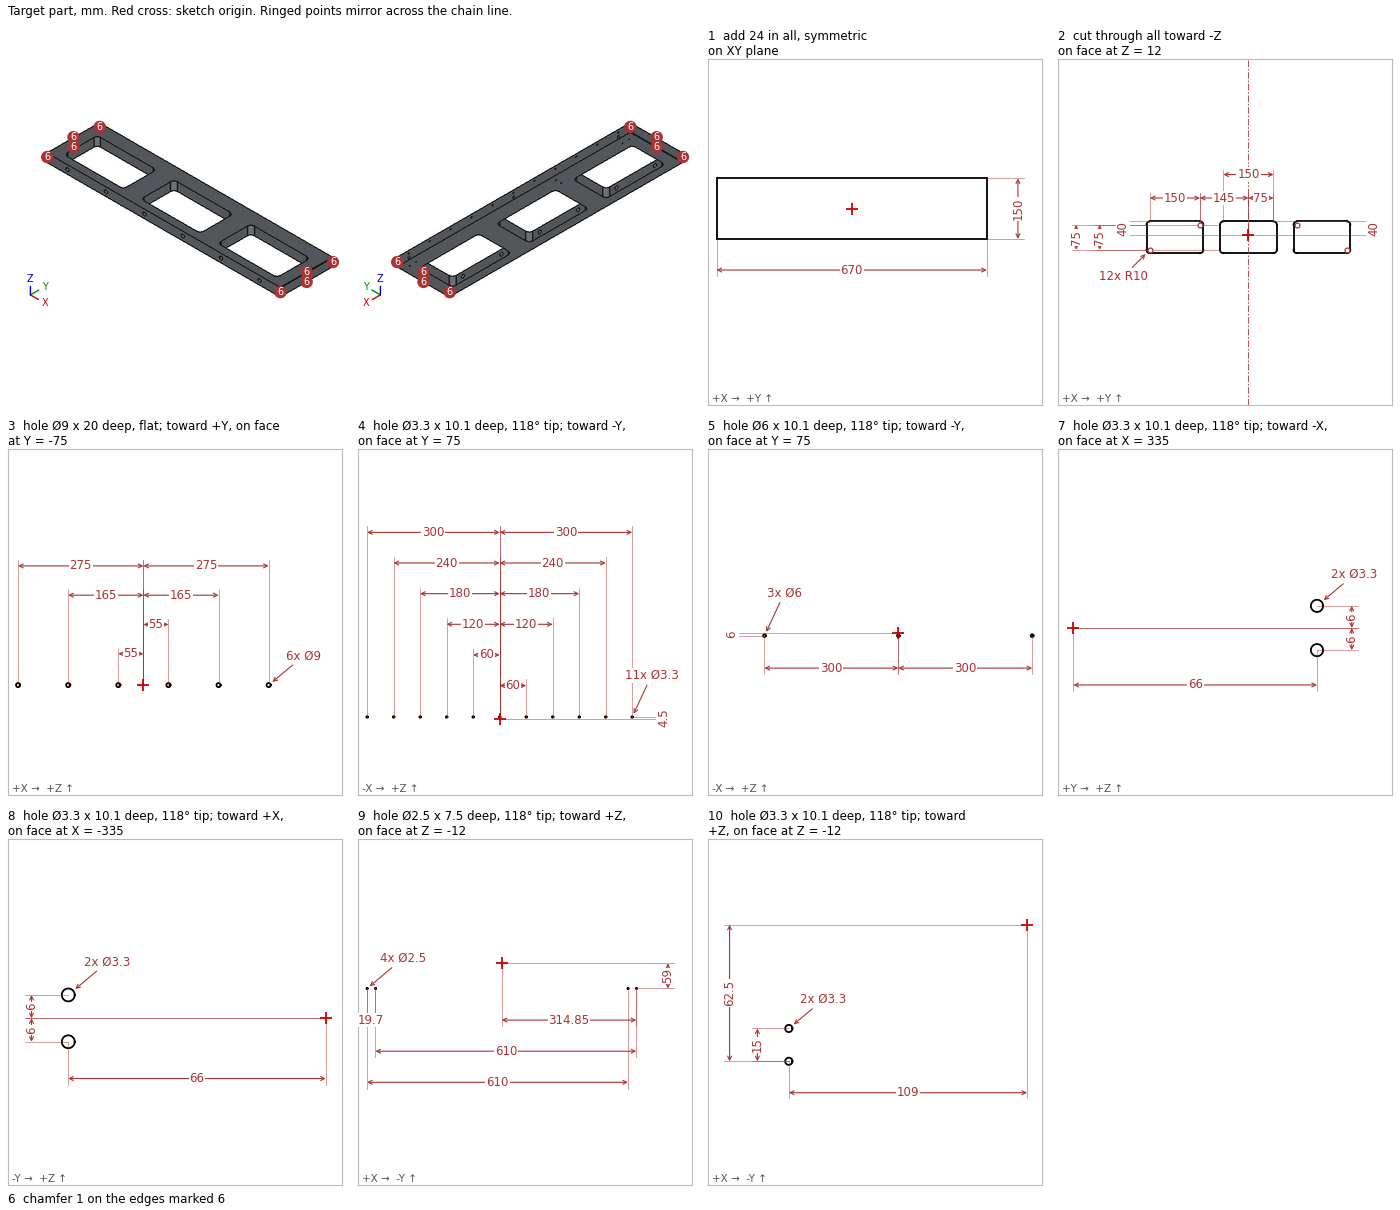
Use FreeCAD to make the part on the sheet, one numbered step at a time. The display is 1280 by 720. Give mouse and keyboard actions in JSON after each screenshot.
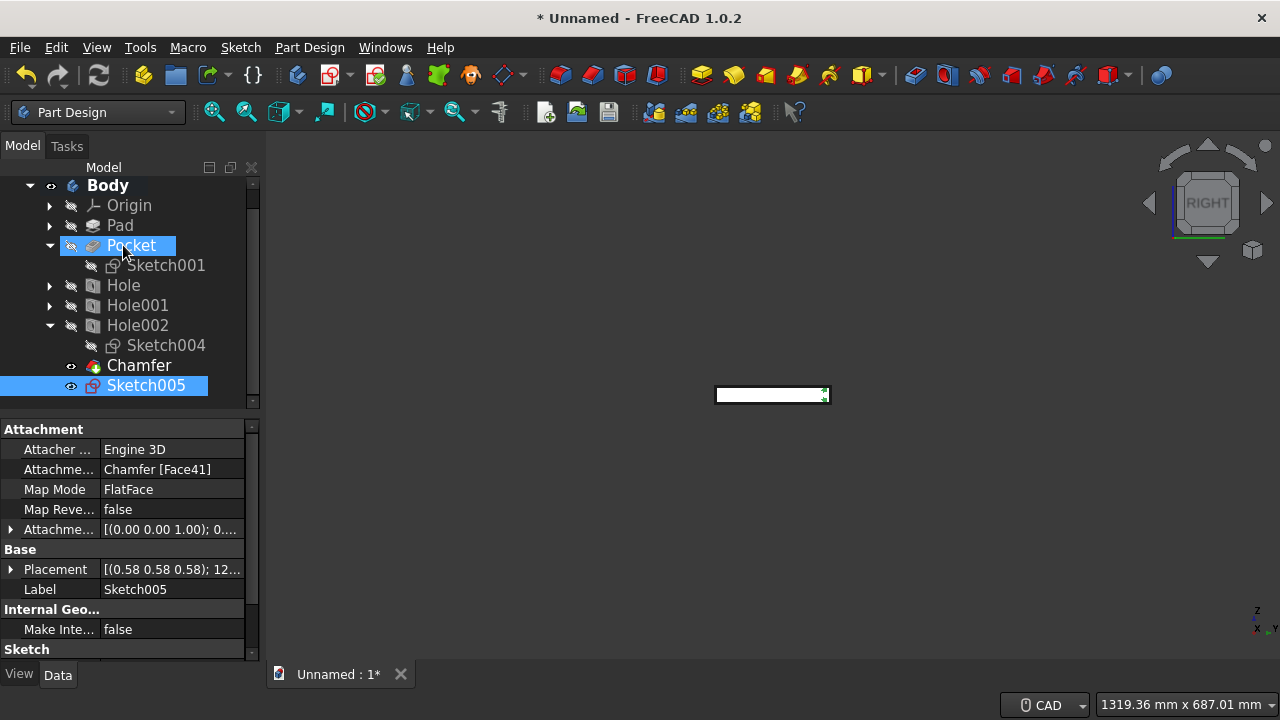
{"action": "left_click", "coordinate": [948, 76]}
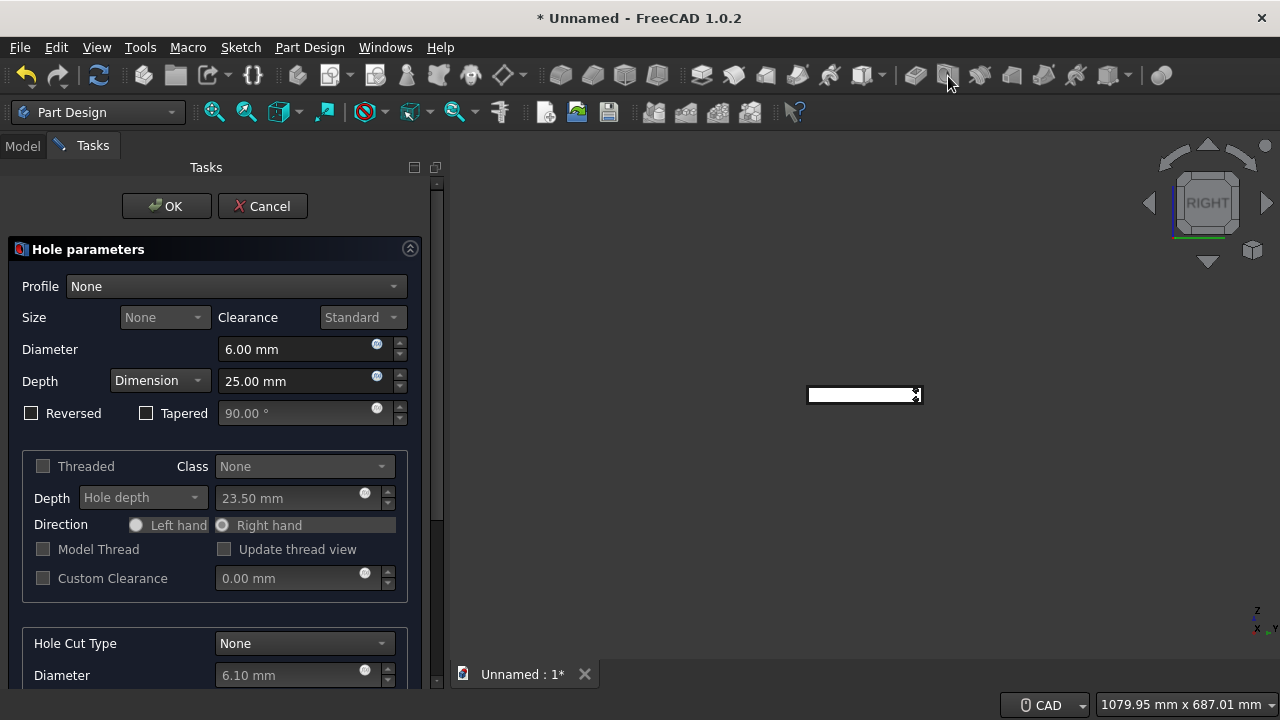
{"action": "triple_click", "coordinate": [305, 349]}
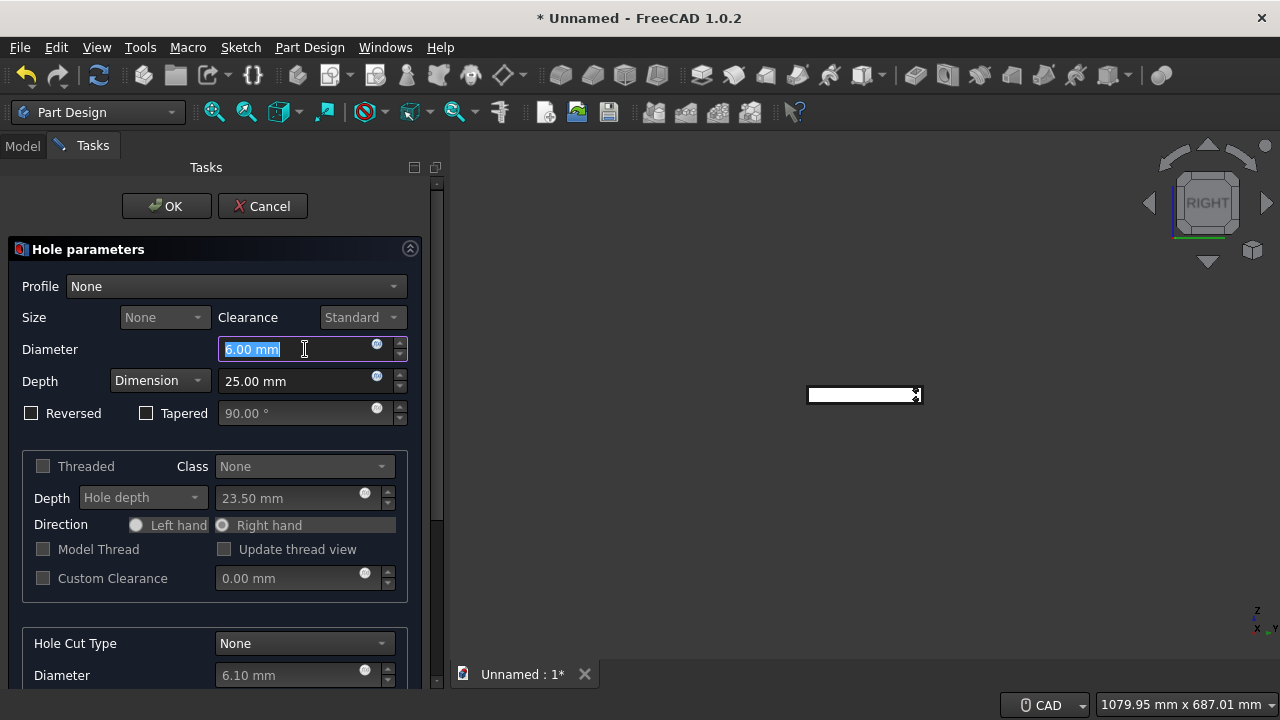
{"action": "type", "text": "3.3"}
{"action": "key", "text": "Tab"}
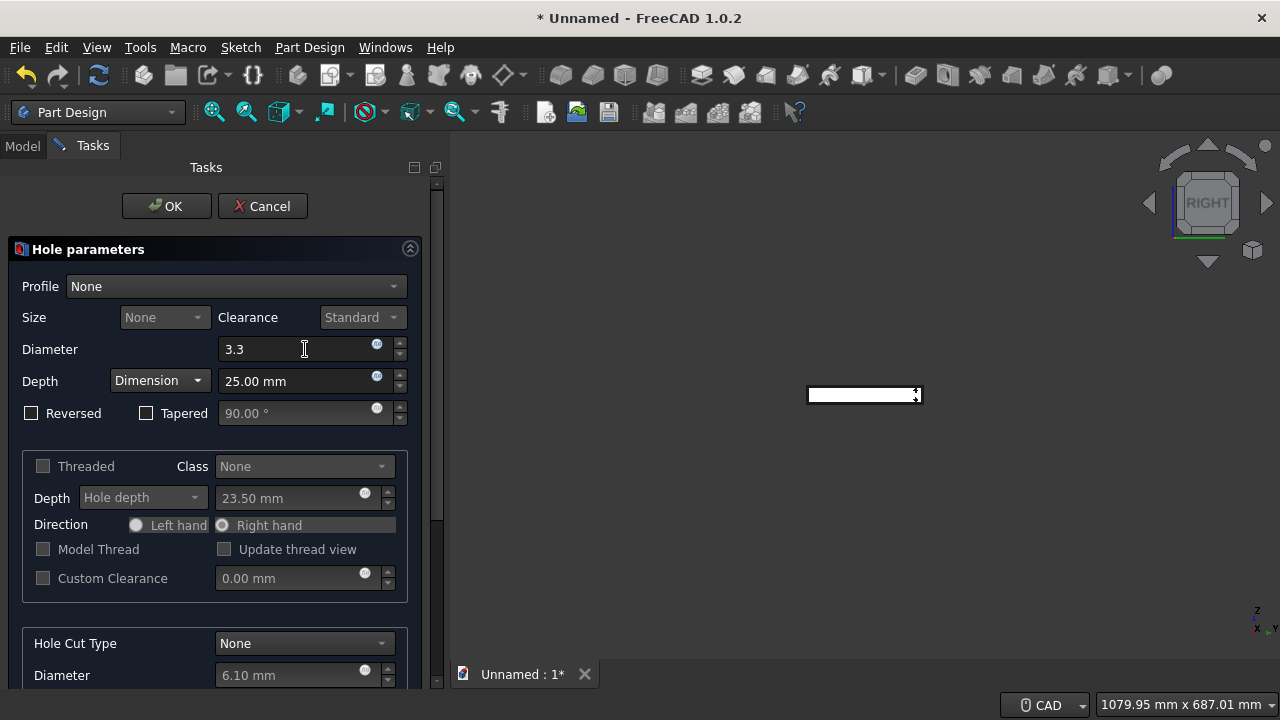
{"action": "triple_click", "coordinate": [305, 381]}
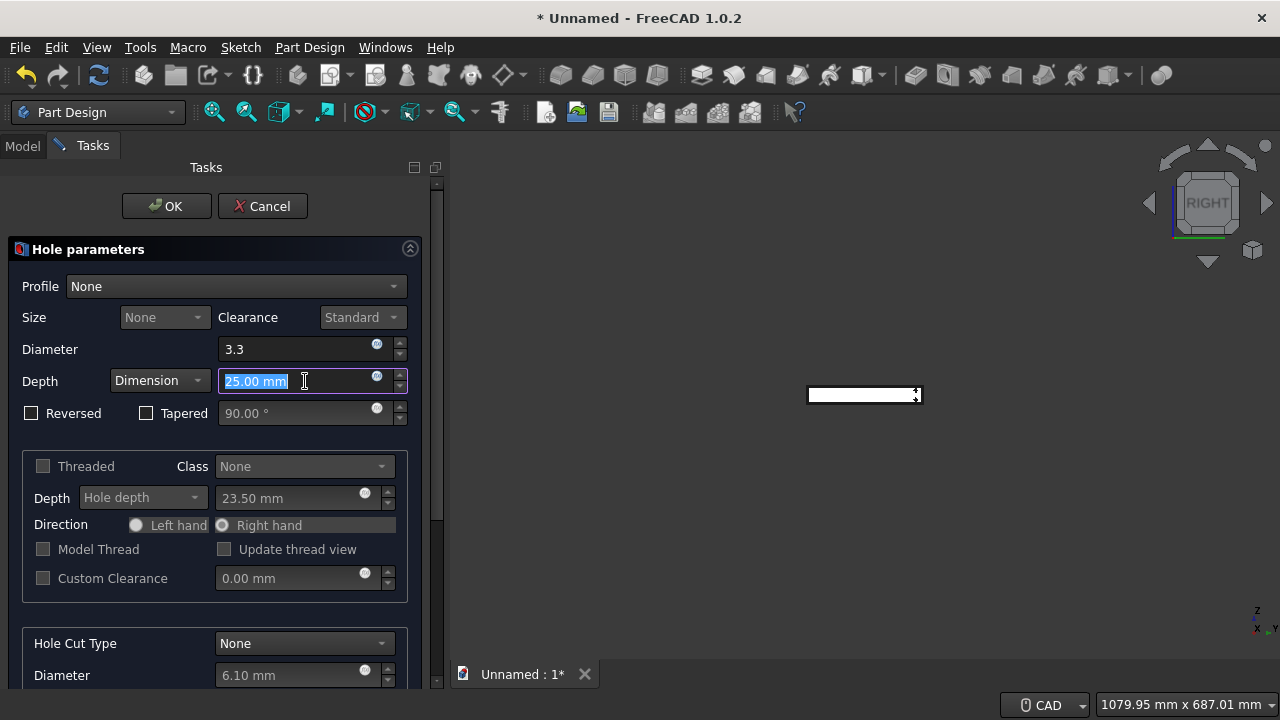
{"action": "type", "text": "10.1"}
{"action": "key", "text": "Tab"}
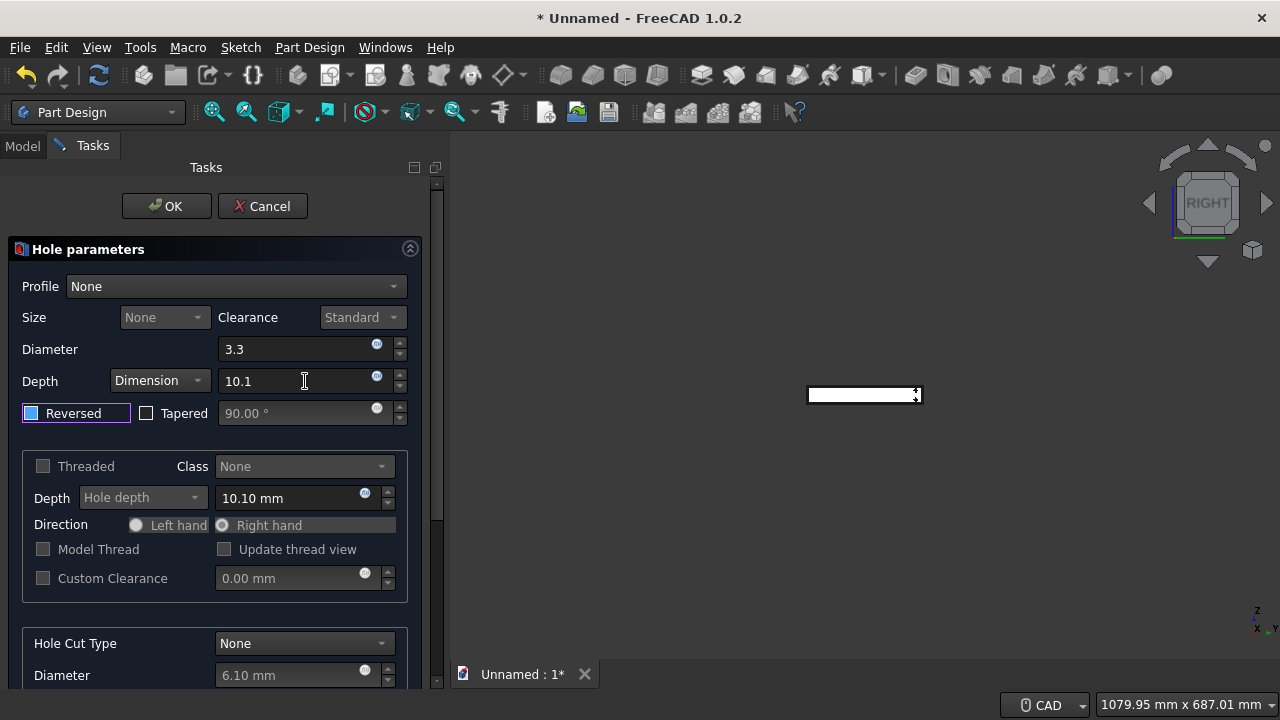
{"action": "left_click", "coordinate": [167, 206]}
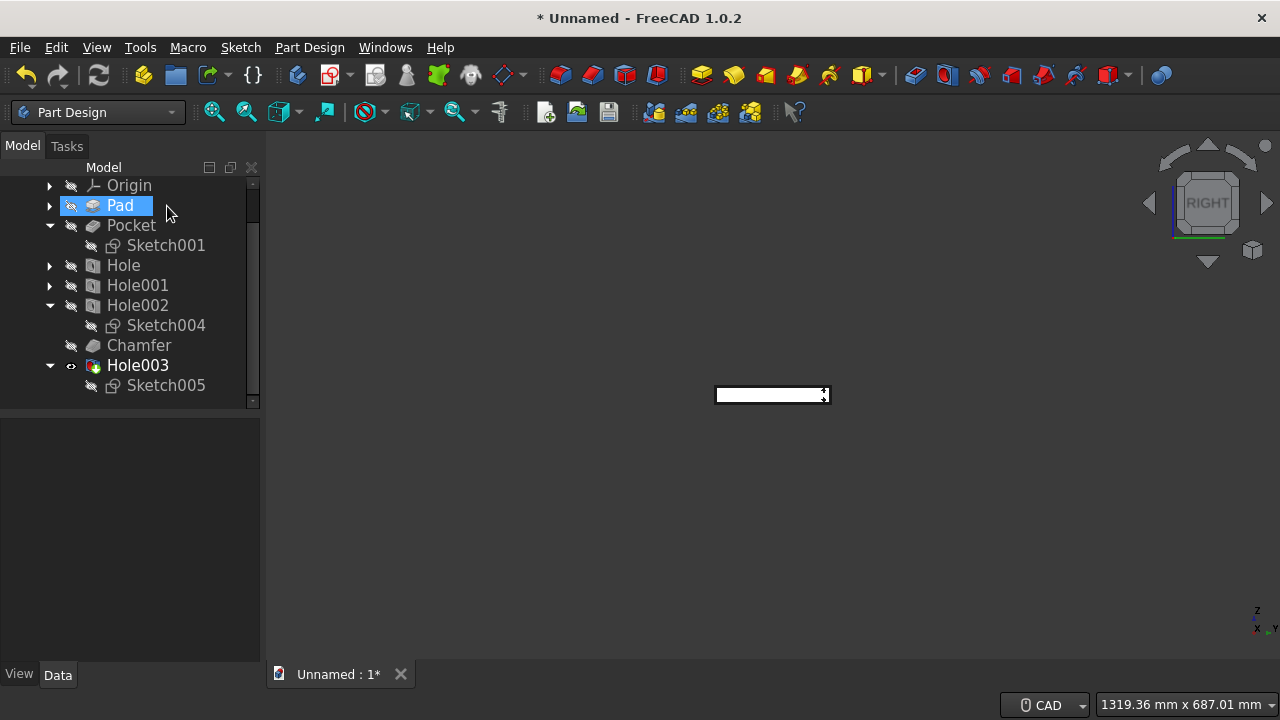
{"action": "left_click", "coordinate": [216, 112]}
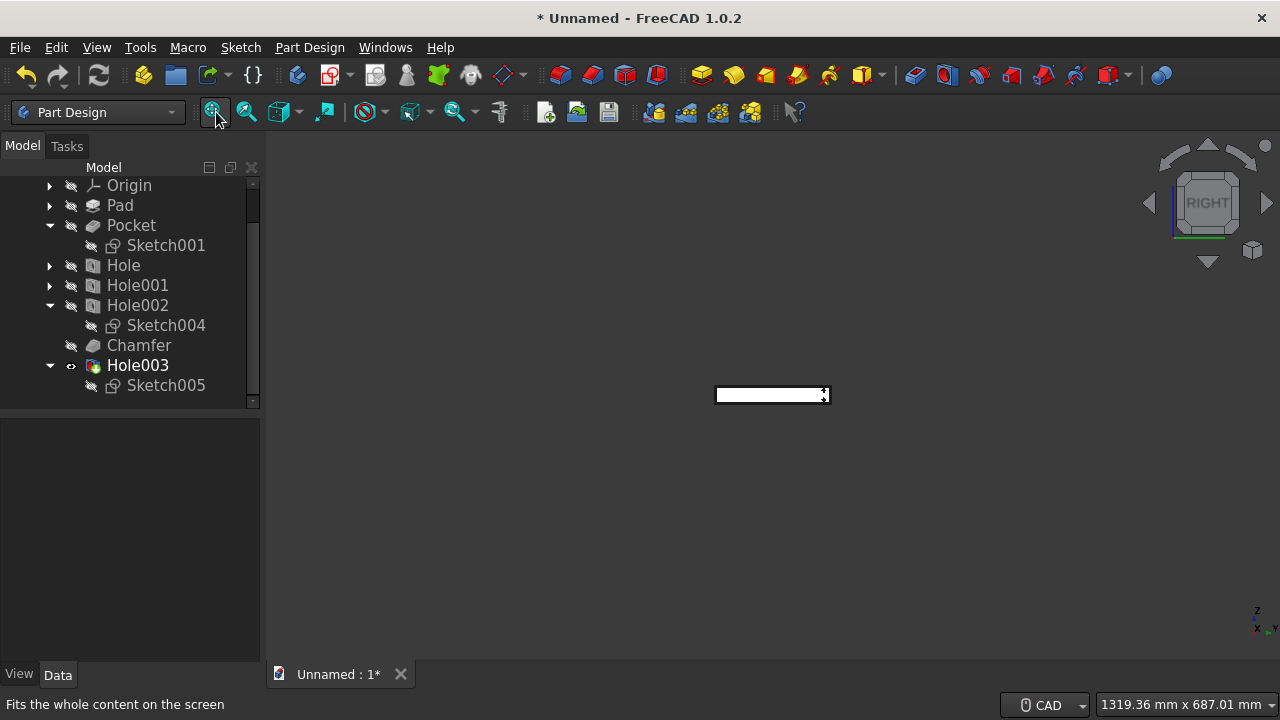
{"action": "key", "text": "6"}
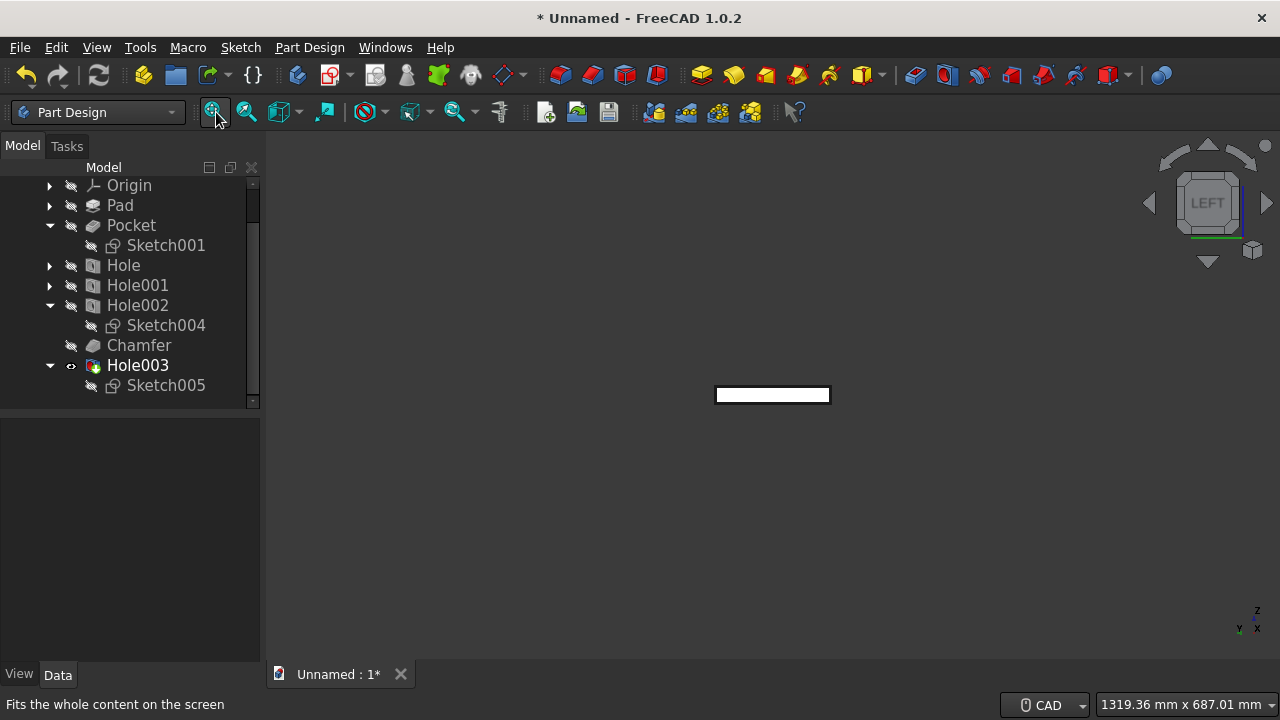
{"action": "key", "text": "v f"}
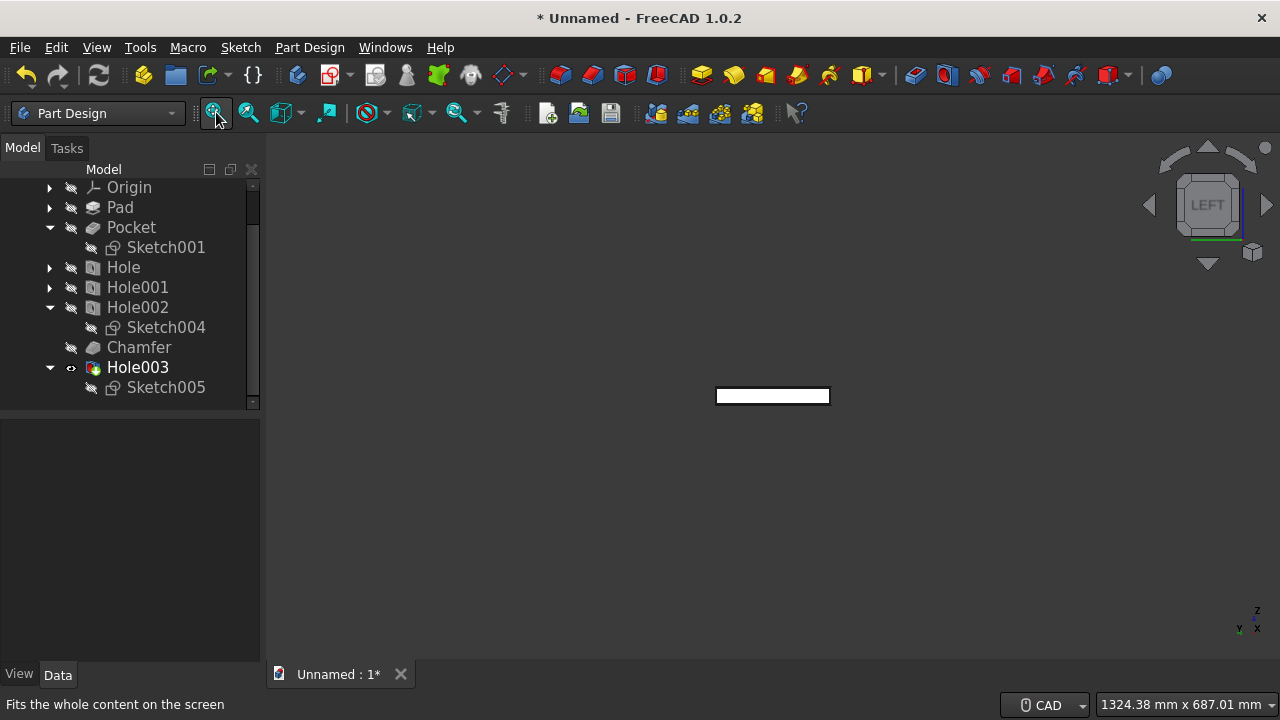
{"action": "left_click", "coordinate": [741, 395]}